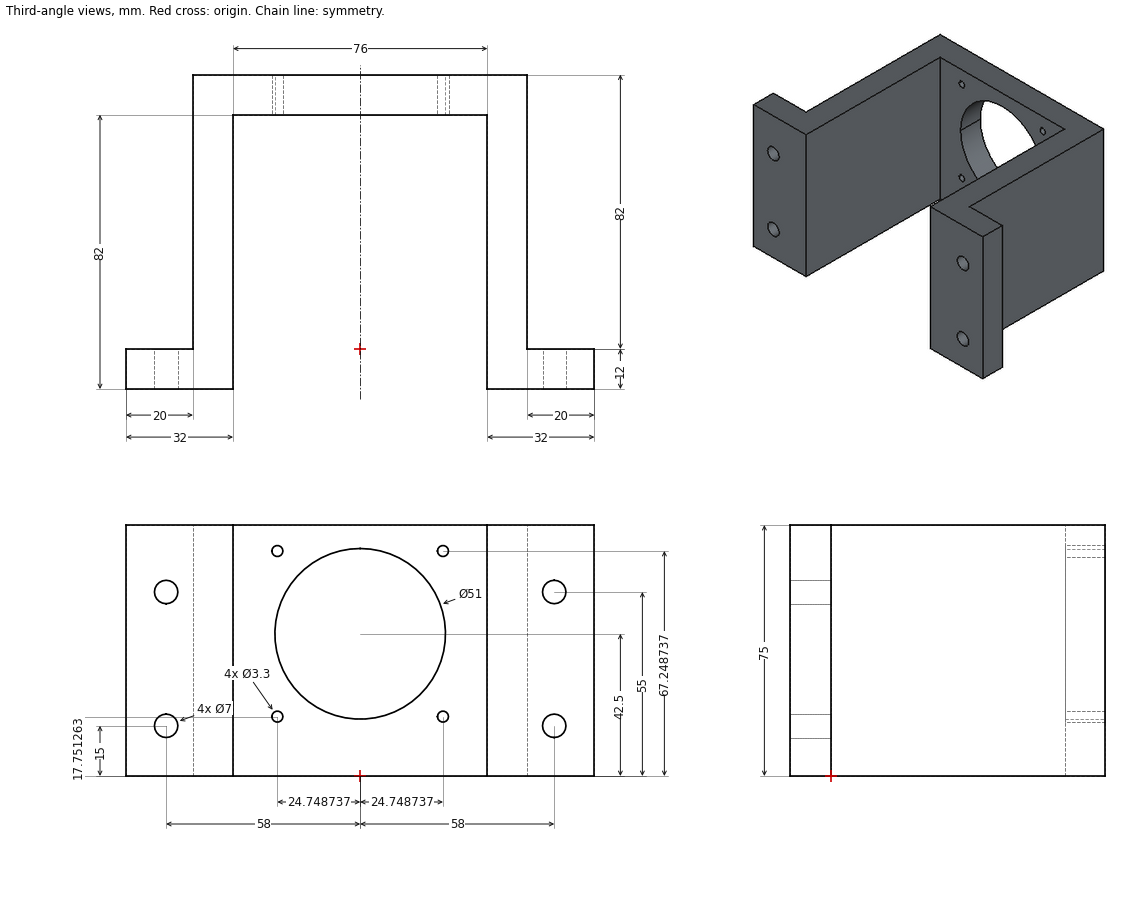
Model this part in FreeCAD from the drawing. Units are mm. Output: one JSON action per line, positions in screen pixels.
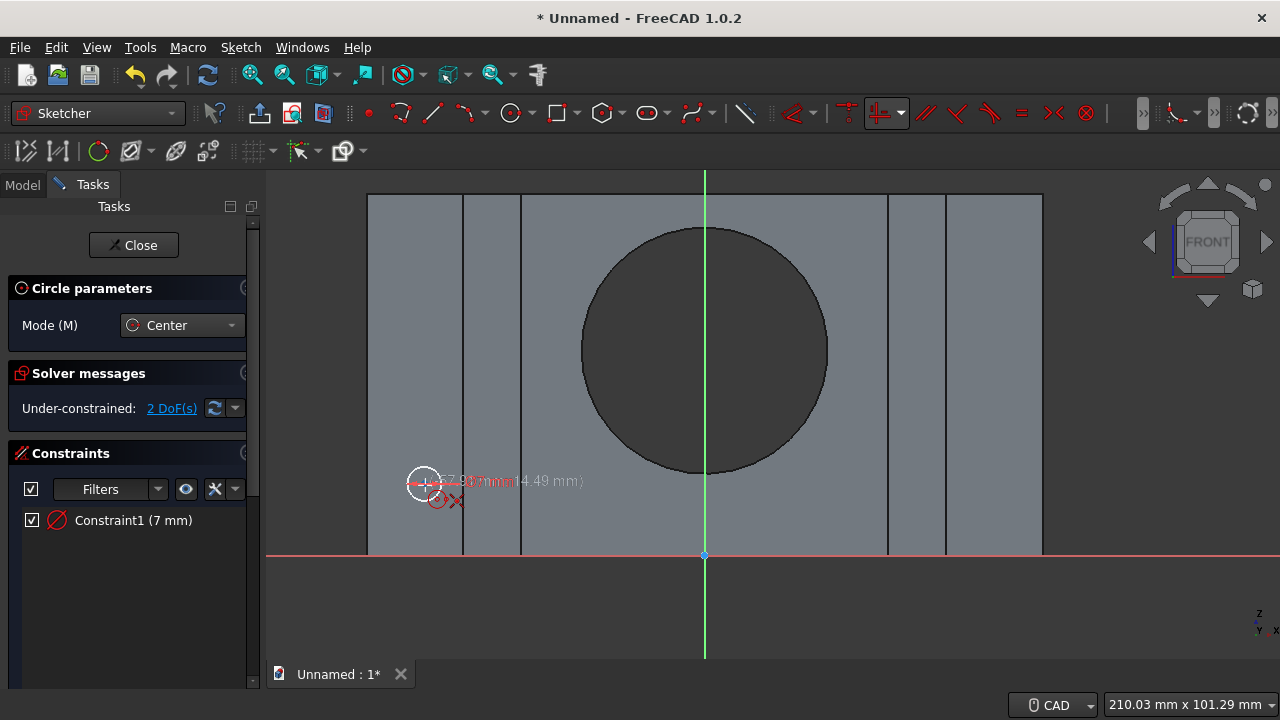
{"action": "scroll", "coordinate": [985, 483], "scroll_direction": "up", "scroll_amount": 2}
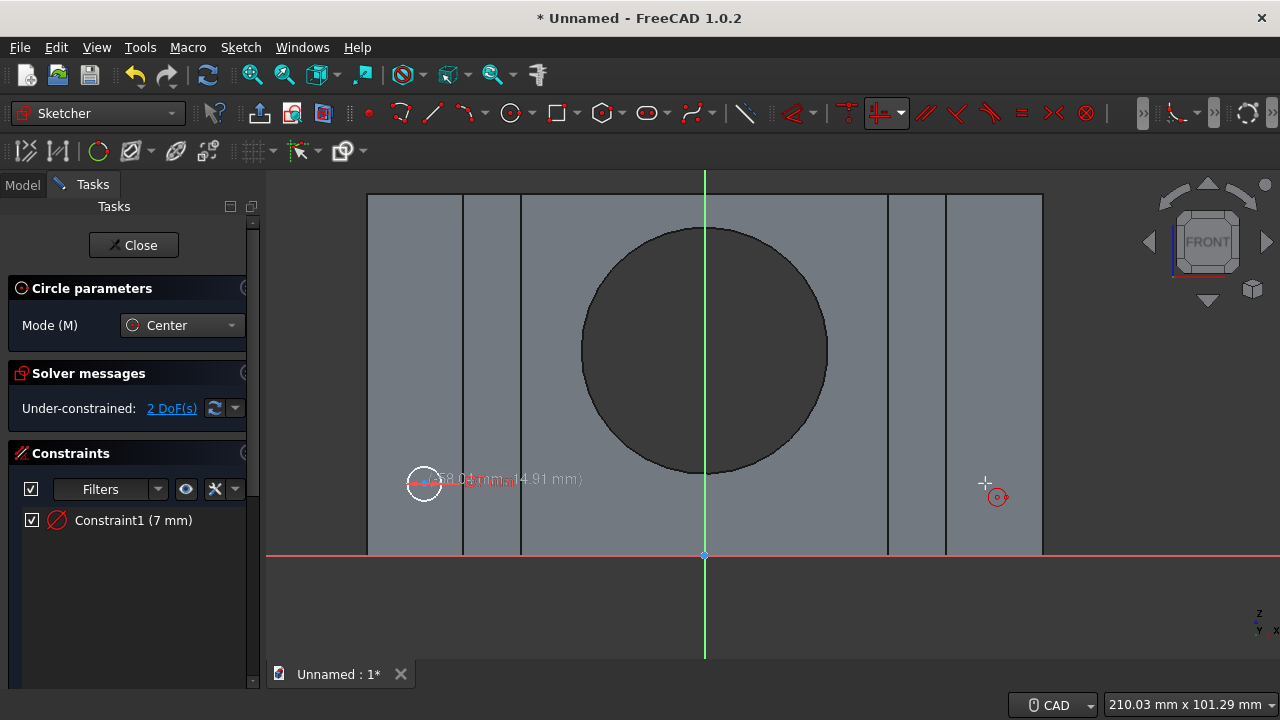
{"action": "left_click", "coordinate": [984, 483]}
{"action": "mouse_move", "coordinate": [1002, 465]}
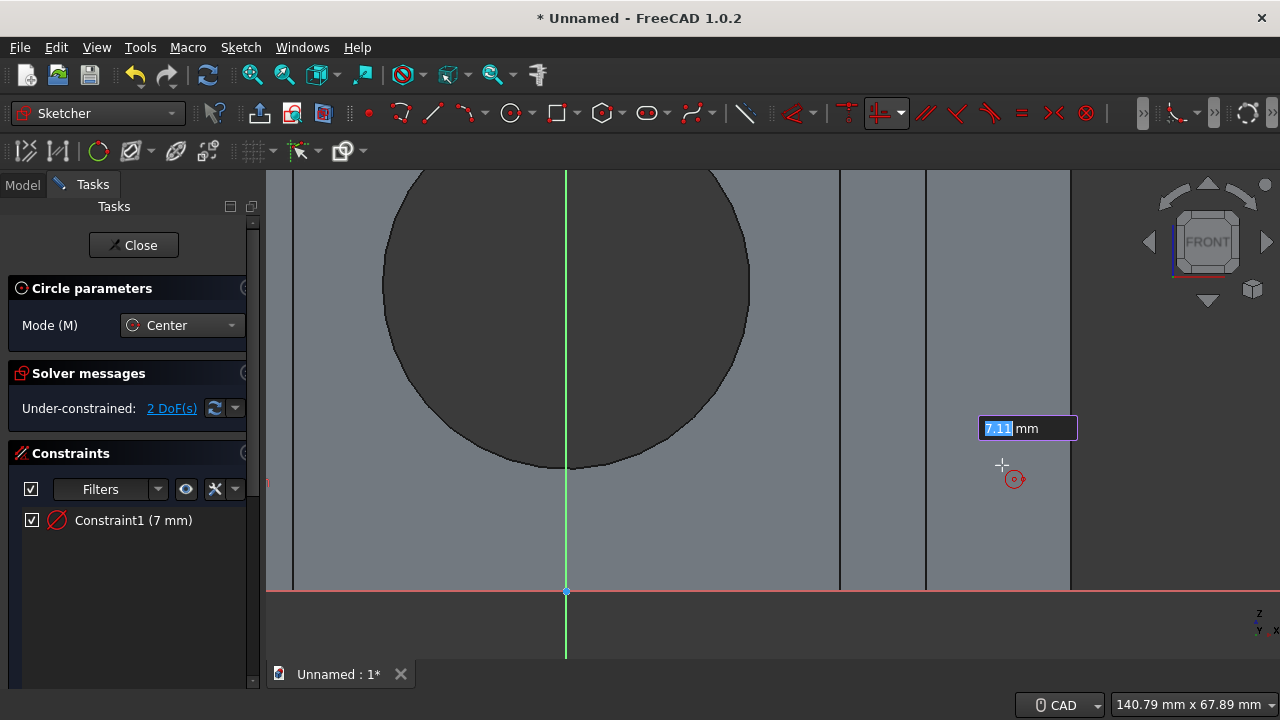
{"action": "type", "text": "7"}
{"action": "key", "text": "Return"}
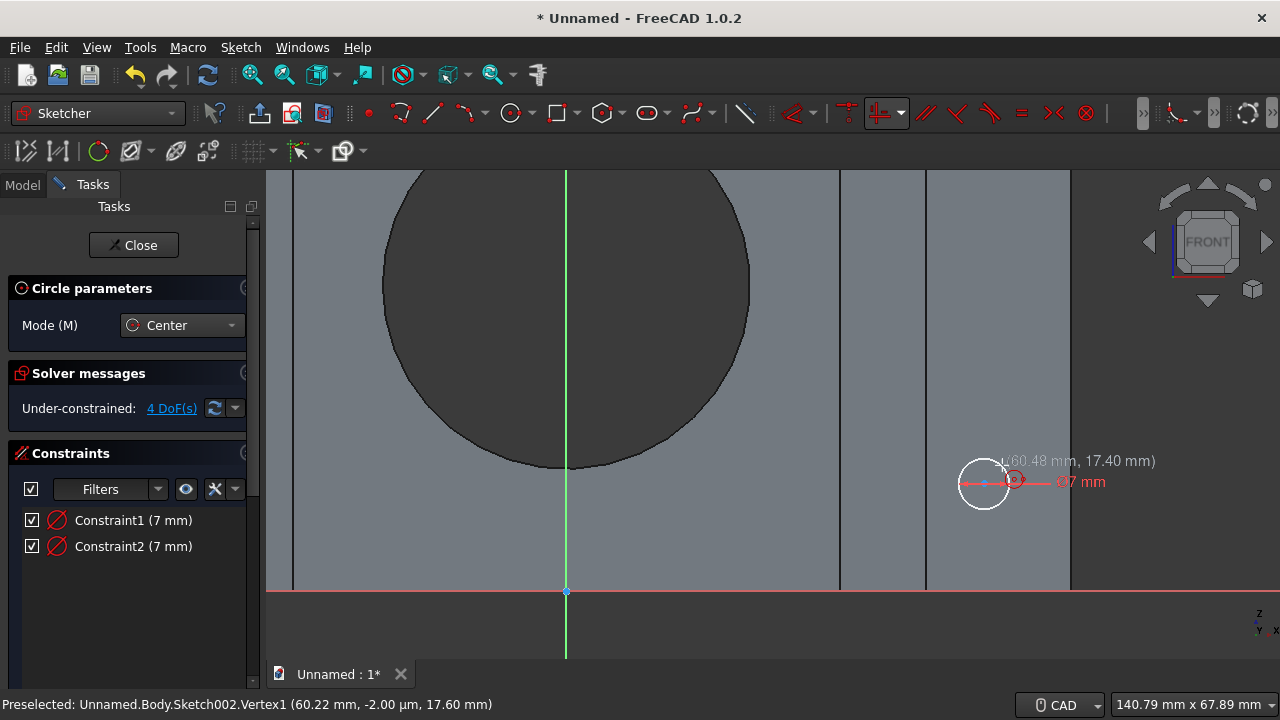
{"action": "scroll", "coordinate": [985, 483], "scroll_direction": "down", "scroll_amount": 2}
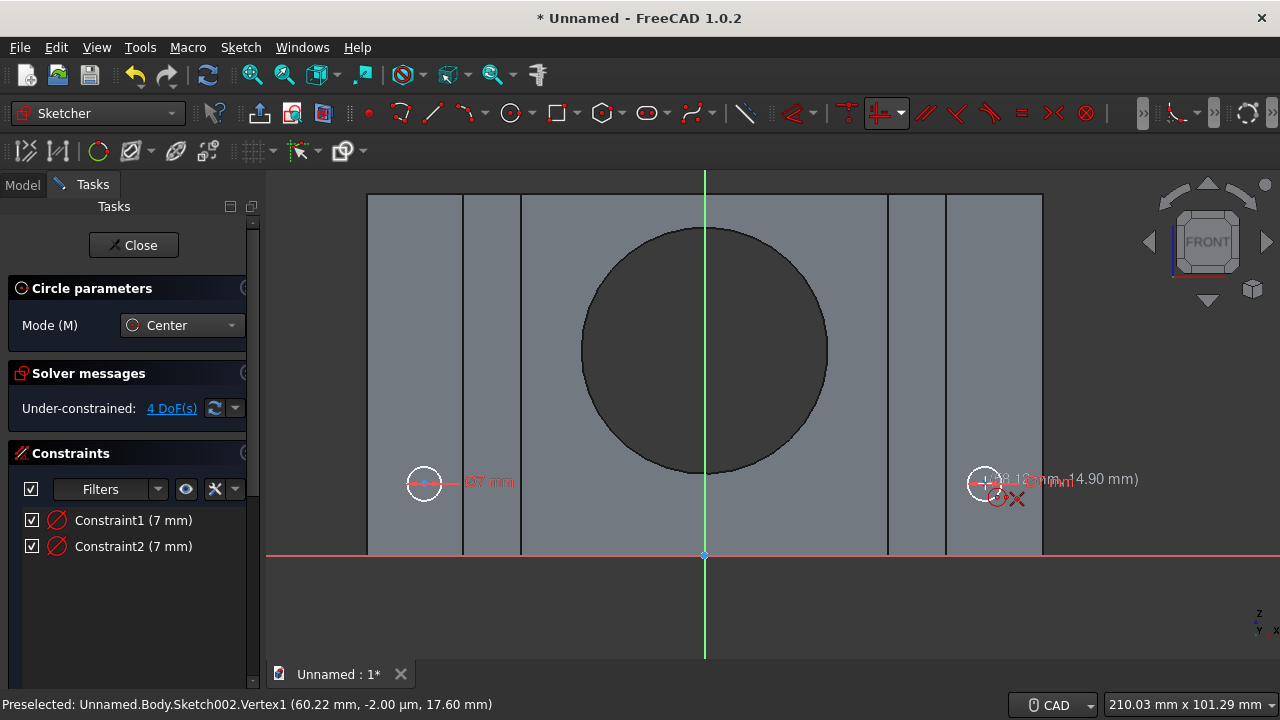
{"action": "scroll", "coordinate": [985, 290], "scroll_direction": "up", "scroll_amount": 2}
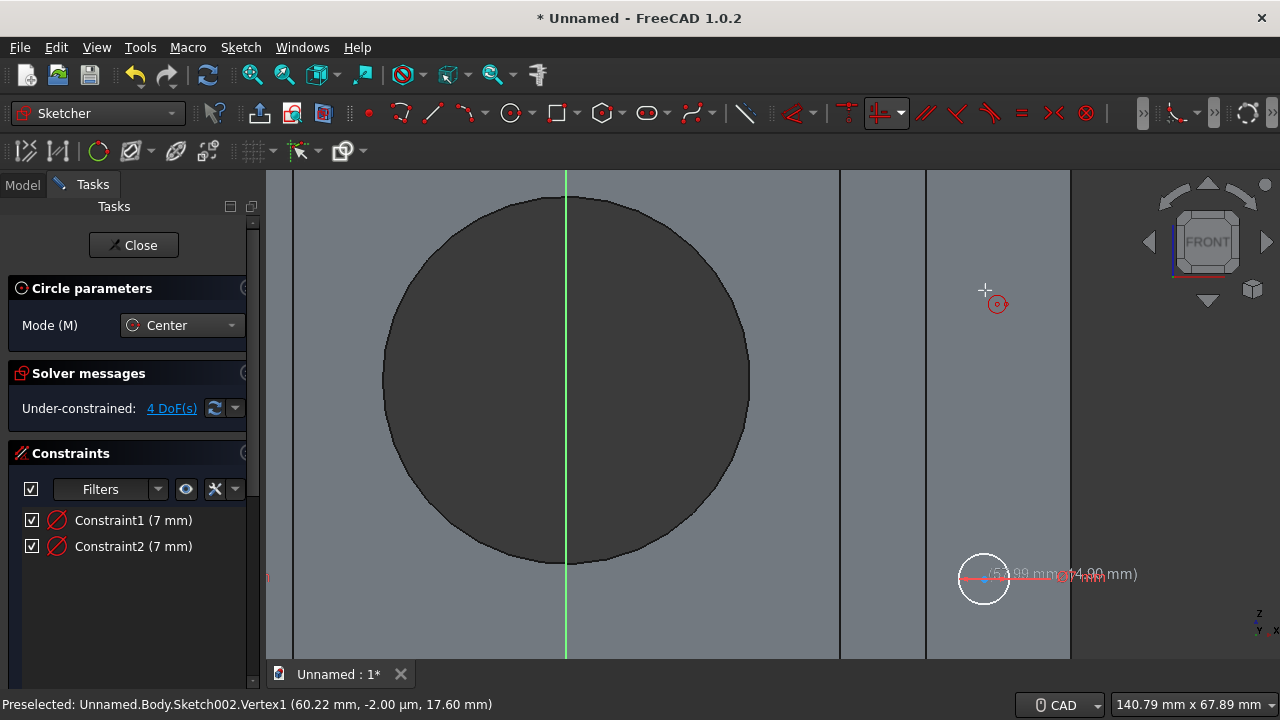
{"action": "left_click", "coordinate": [984, 290]}
{"action": "mouse_move", "coordinate": [1002, 273]}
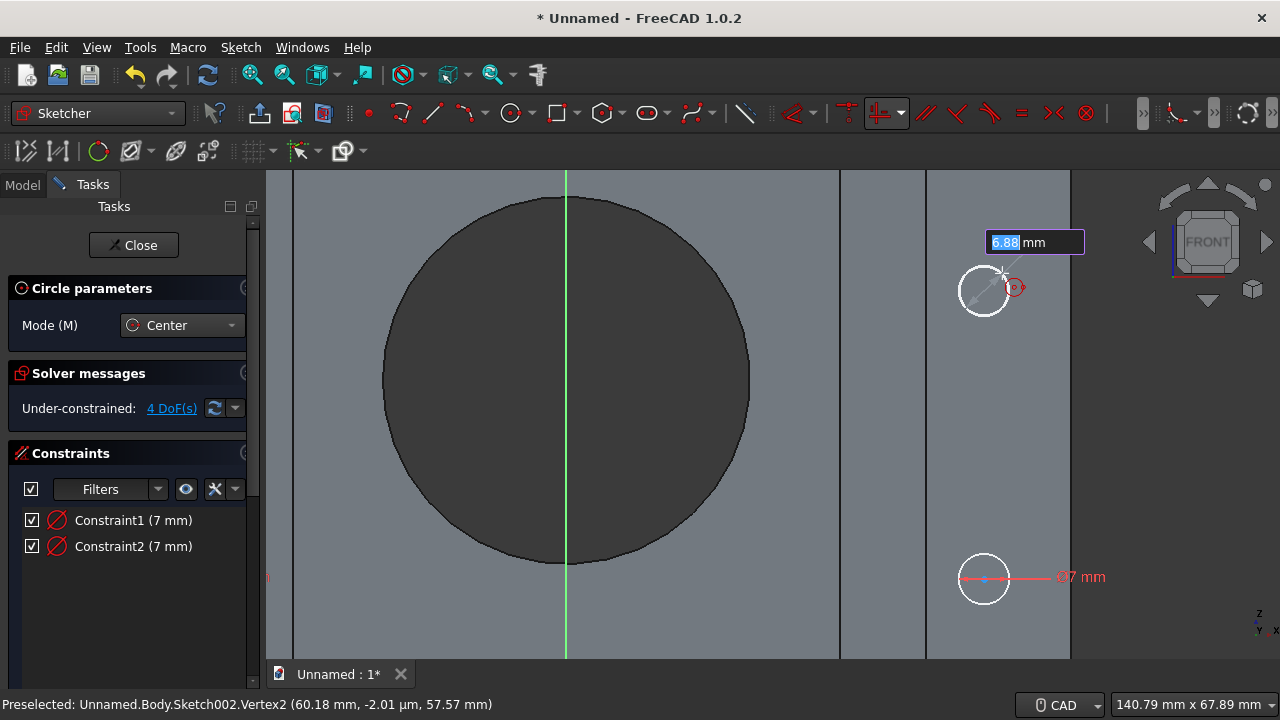
{"action": "type", "text": "7"}
{"action": "key", "text": "Return"}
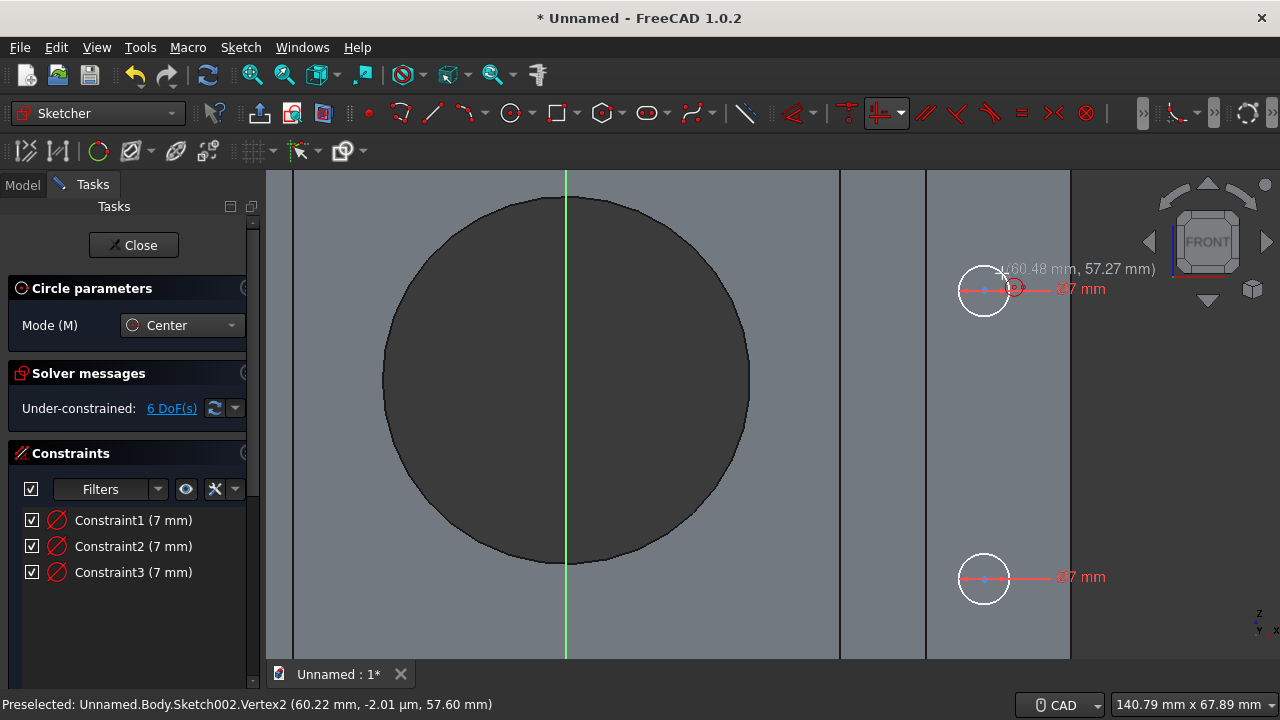
{"action": "scroll", "coordinate": [985, 290], "scroll_direction": "down", "scroll_amount": 2}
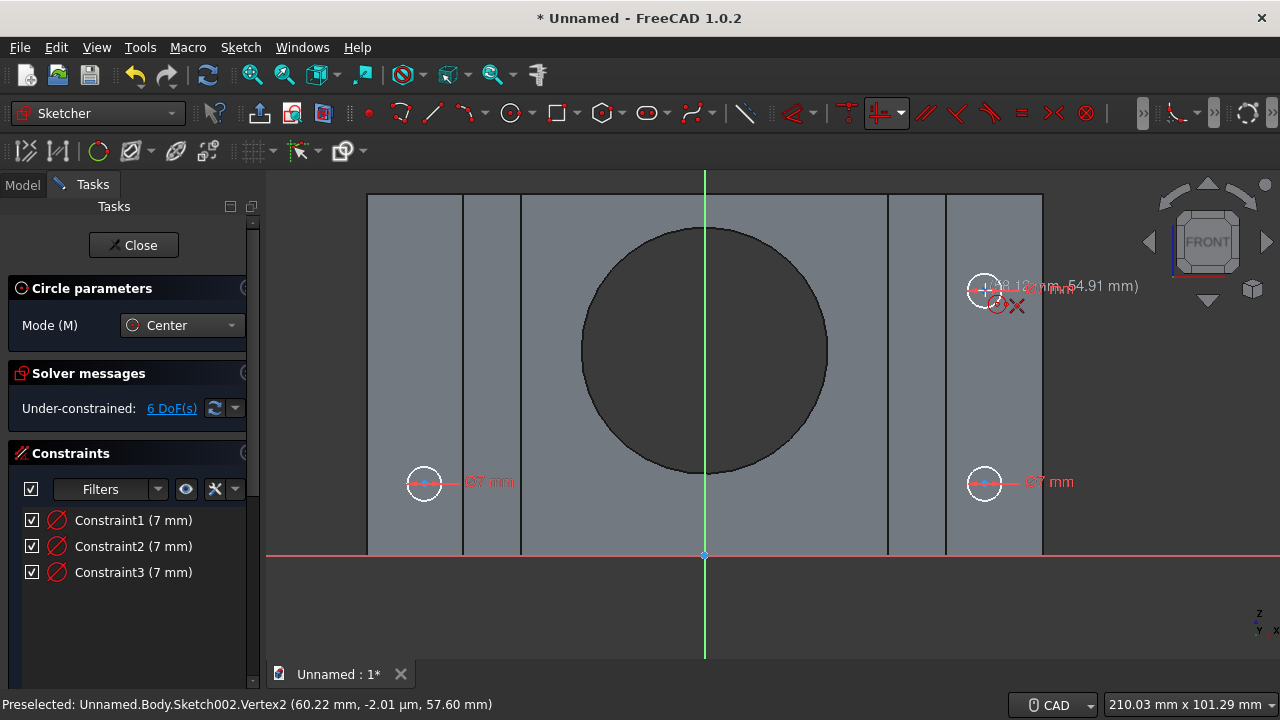
{"action": "scroll", "coordinate": [425, 290], "scroll_direction": "up", "scroll_amount": 2}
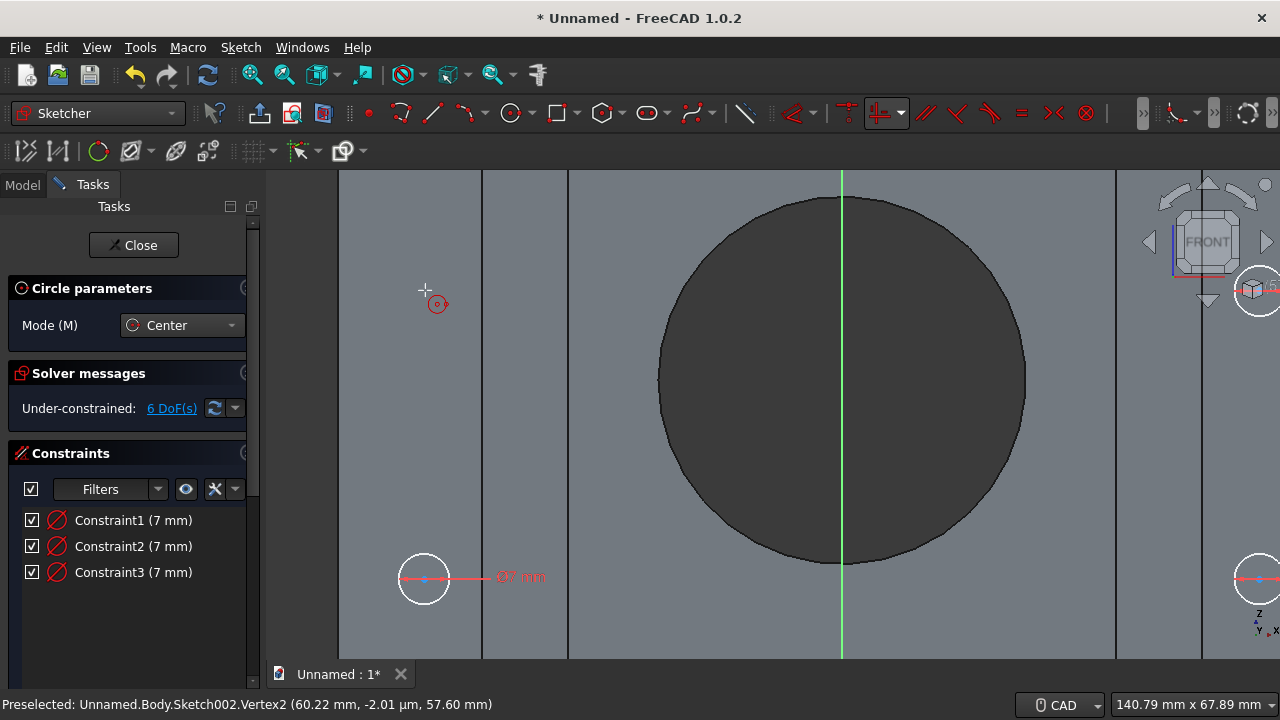
{"action": "left_click", "coordinate": [424, 290]}
{"action": "mouse_move", "coordinate": [442, 273]}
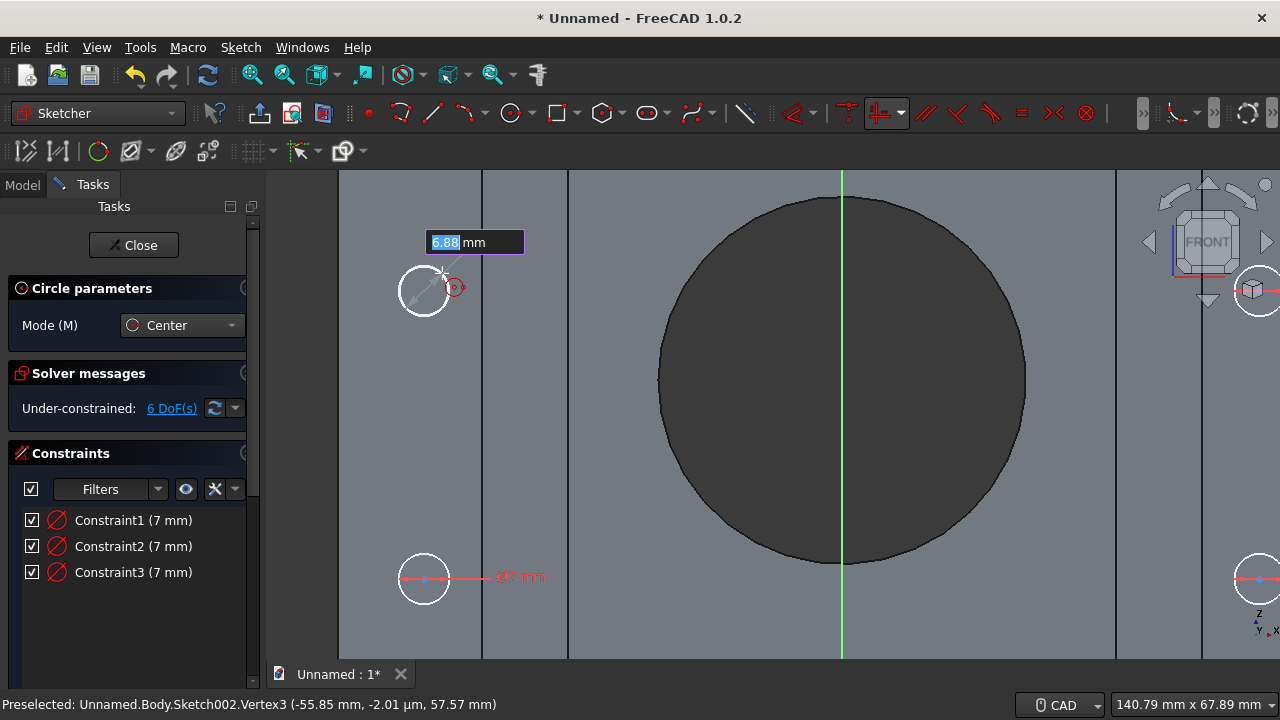
{"action": "type", "text": "7"}
{"action": "key", "text": "Return"}
{"action": "key", "text": "Escape"}